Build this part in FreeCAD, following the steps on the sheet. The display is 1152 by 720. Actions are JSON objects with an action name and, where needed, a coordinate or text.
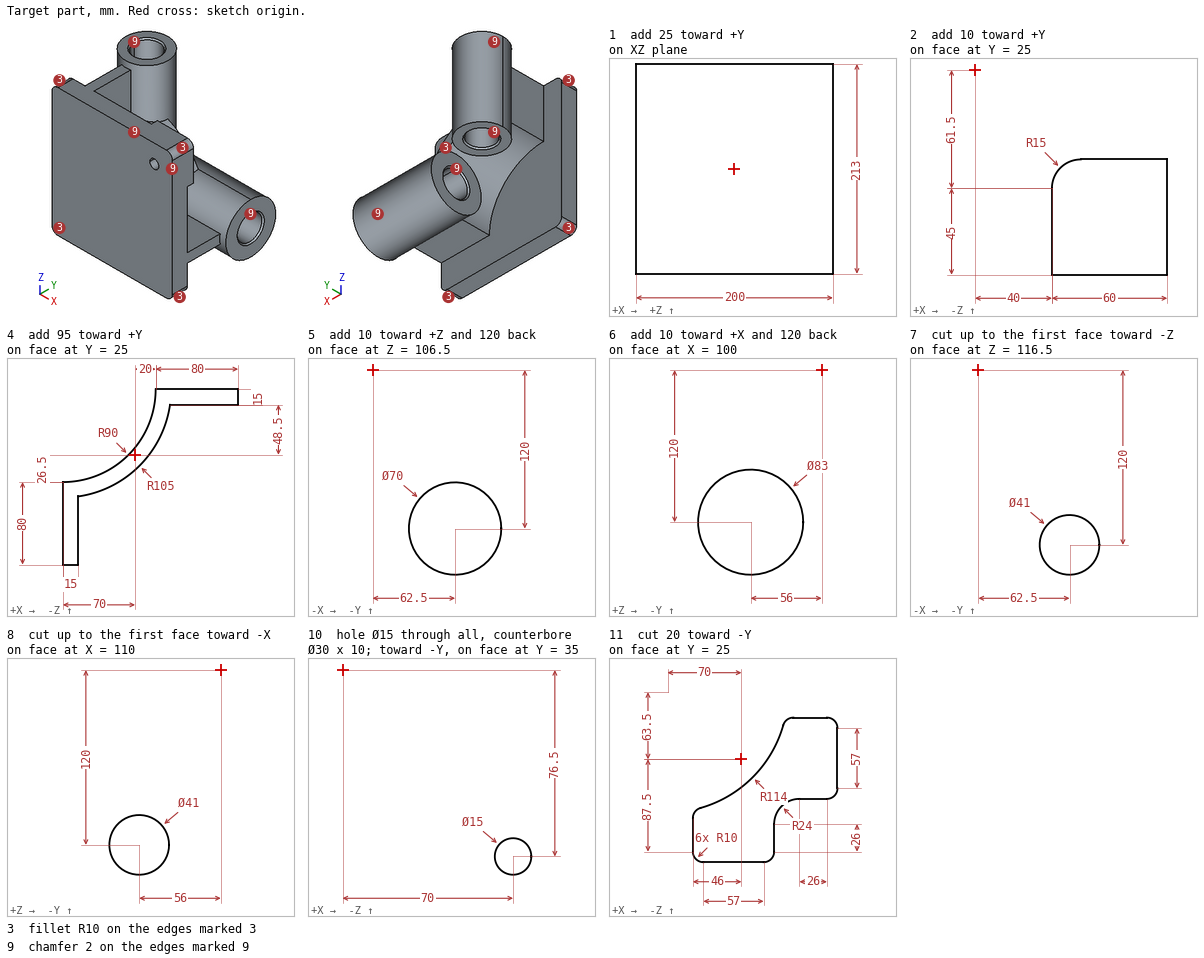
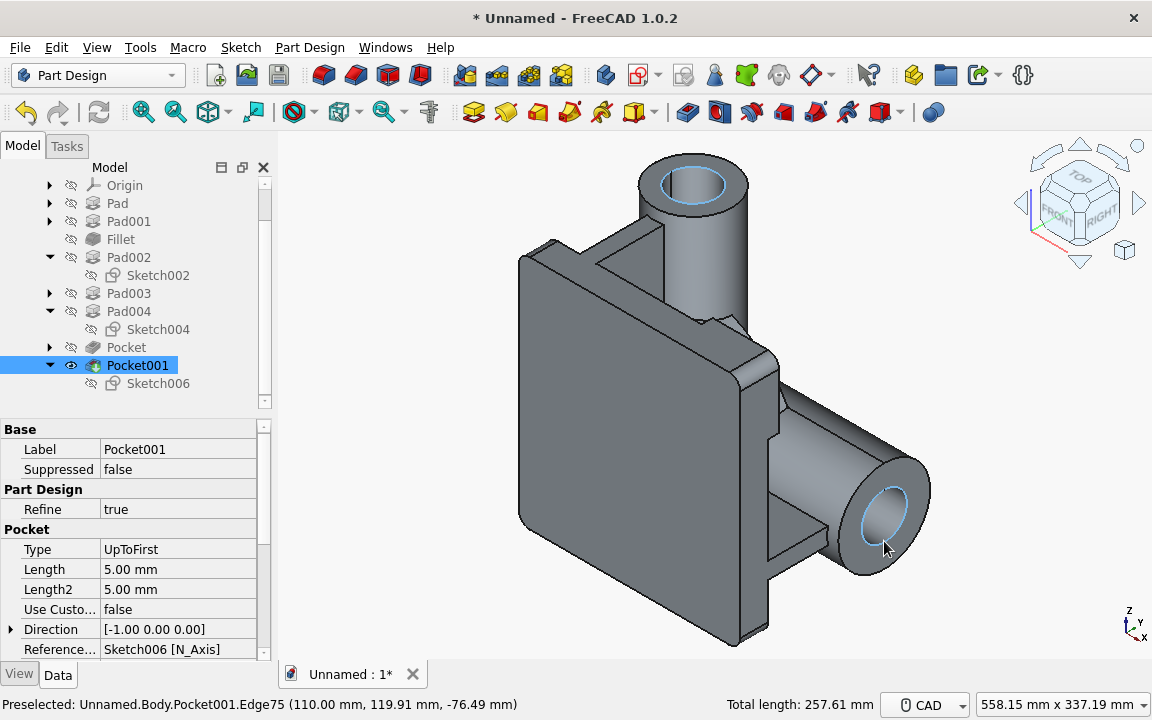
{"action": "key", "text": "2"}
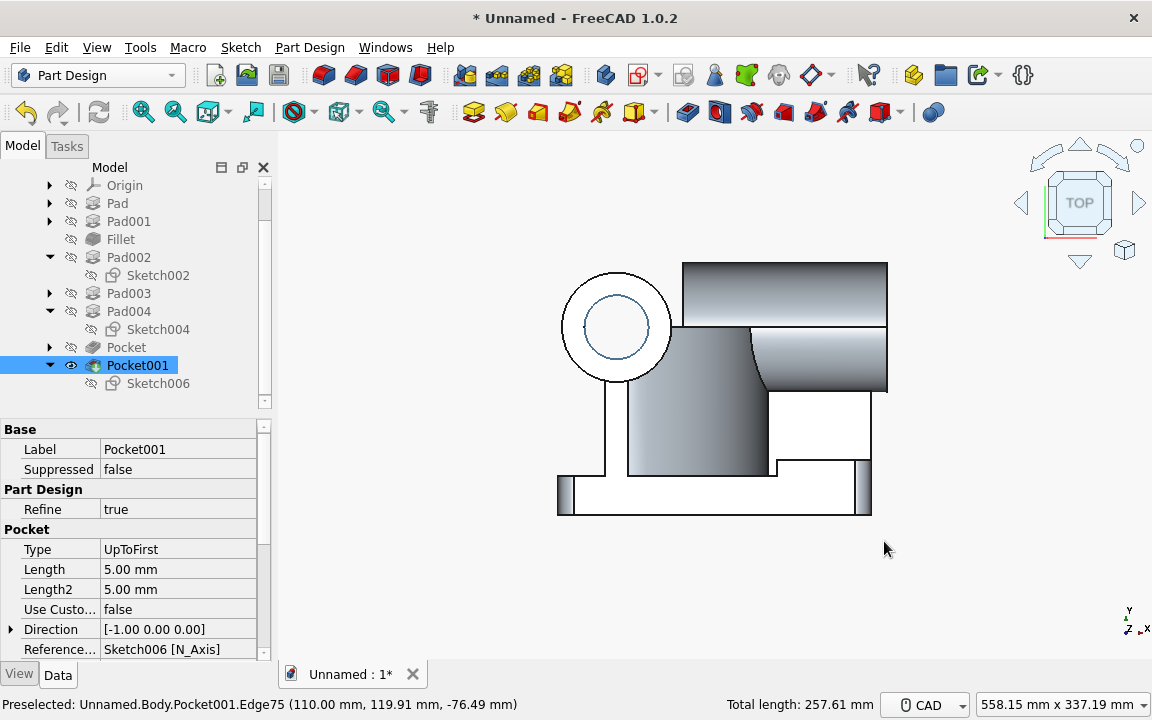
{"action": "key", "text": "0"}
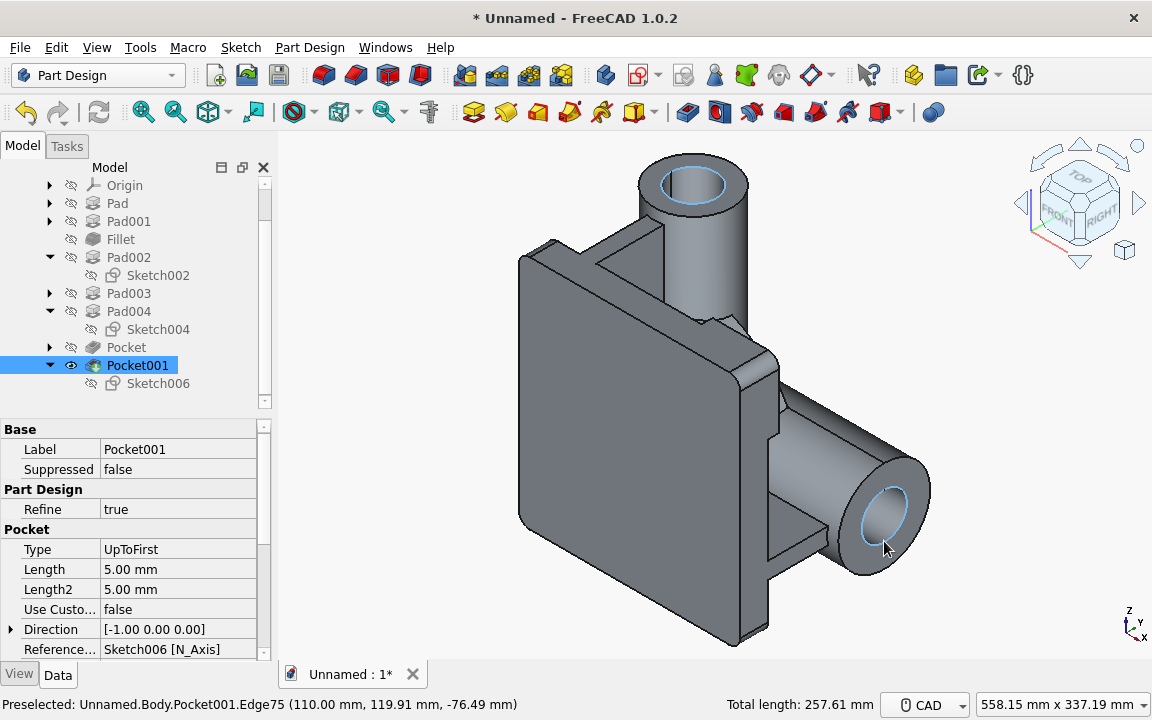
{"action": "key", "text": "1"}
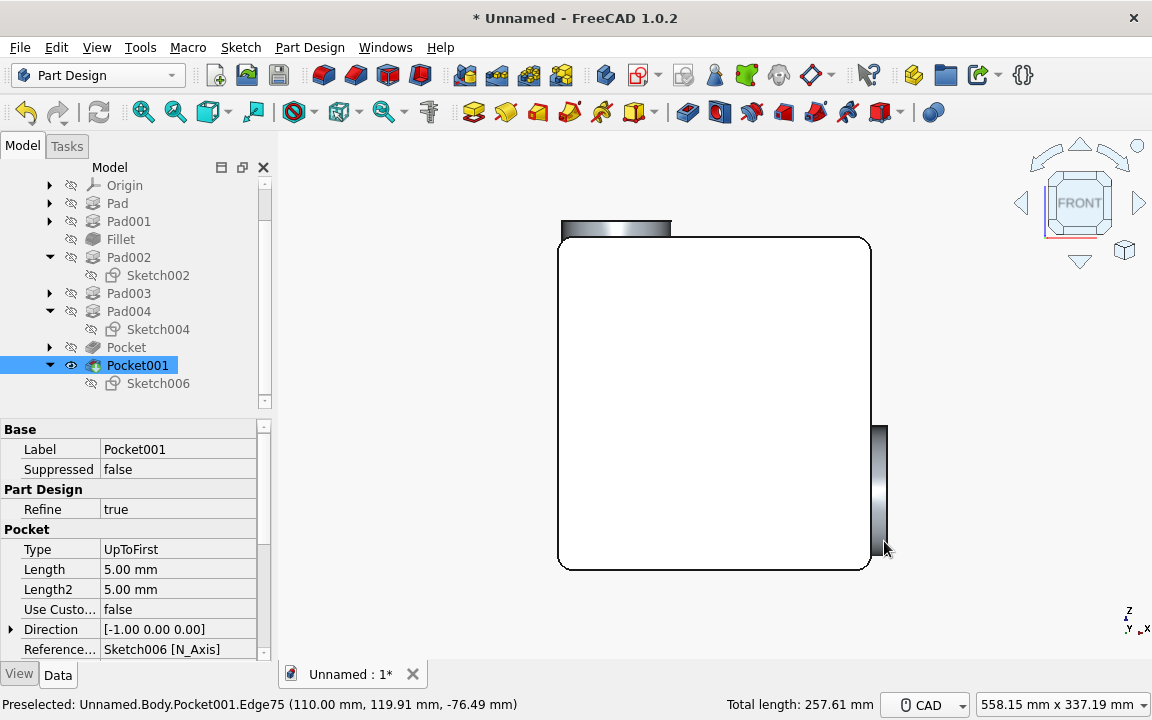
{"action": "key", "text": "3"}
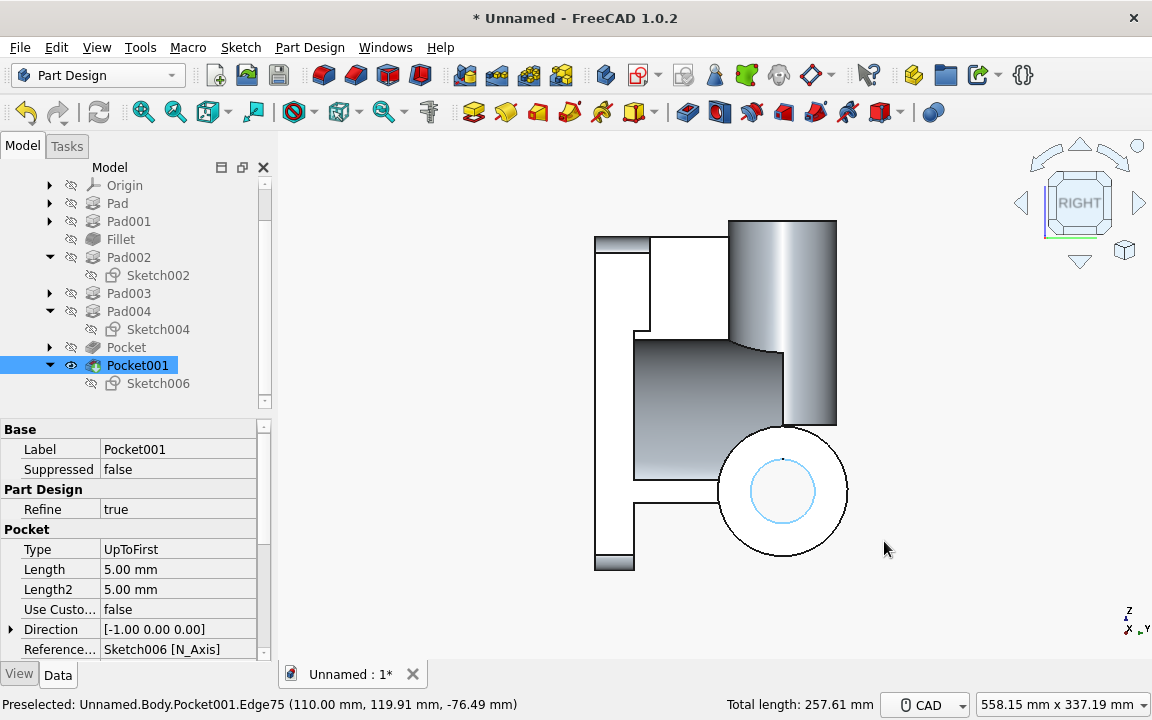
{"action": "key", "text": "5"}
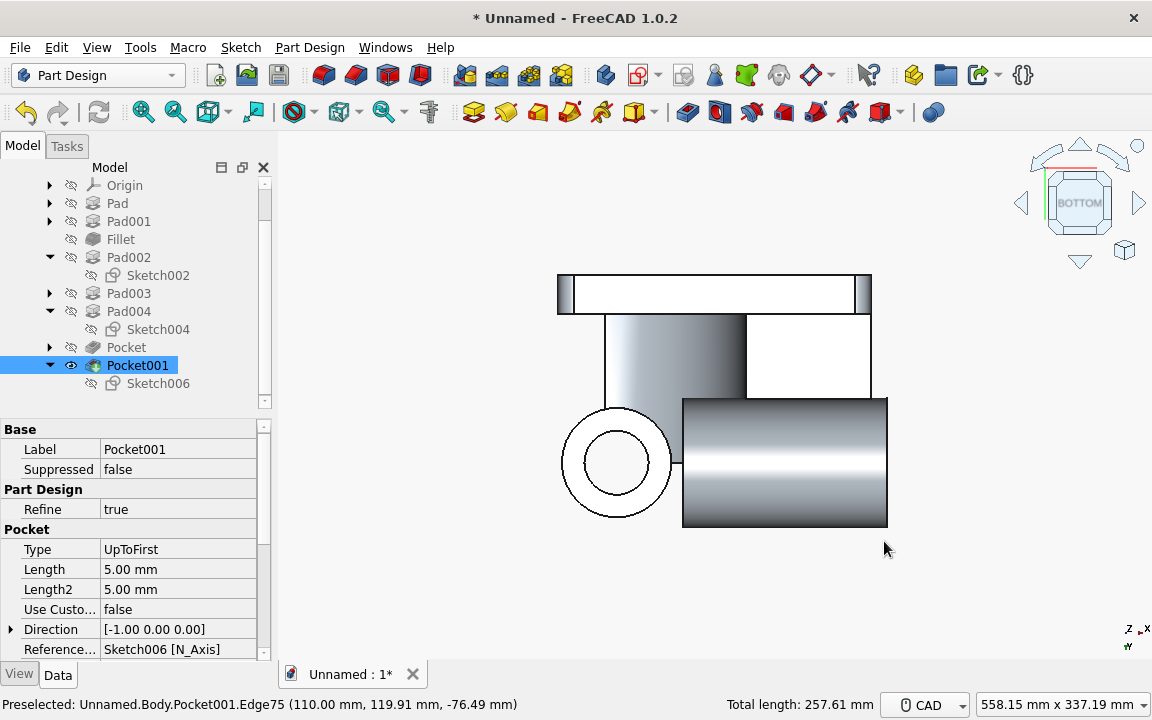
{"action": "left_click", "coordinate": [643, 443], "text": "ctrl"}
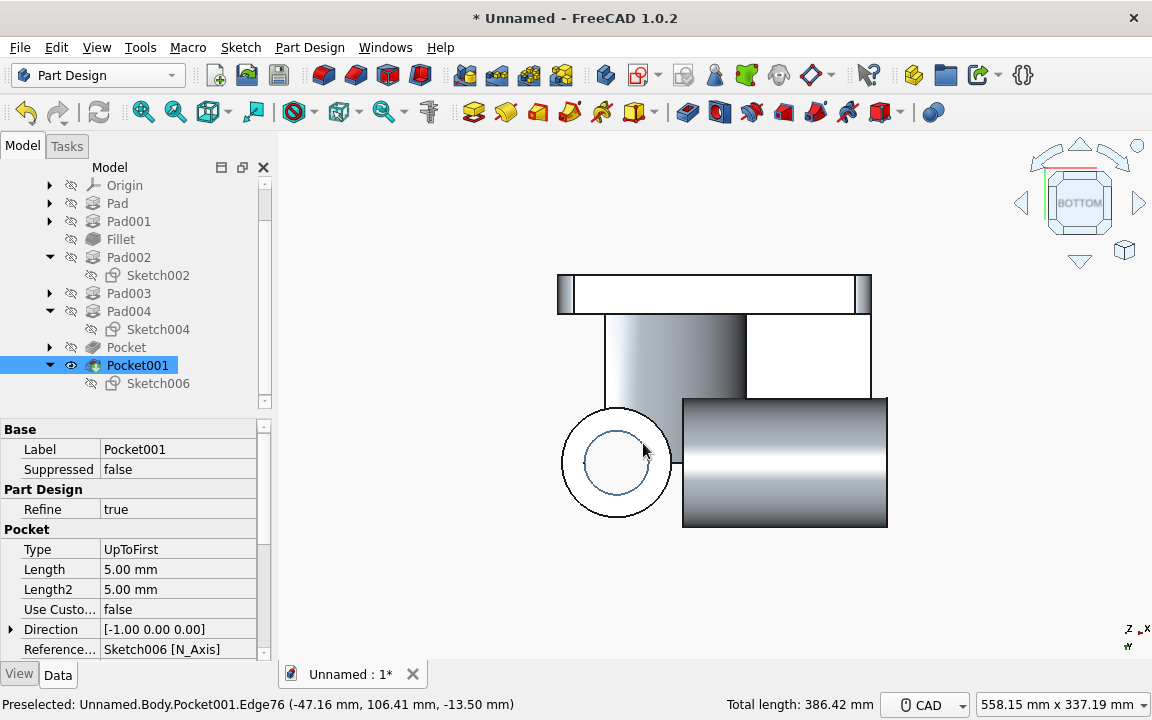
{"action": "key", "text": "4"}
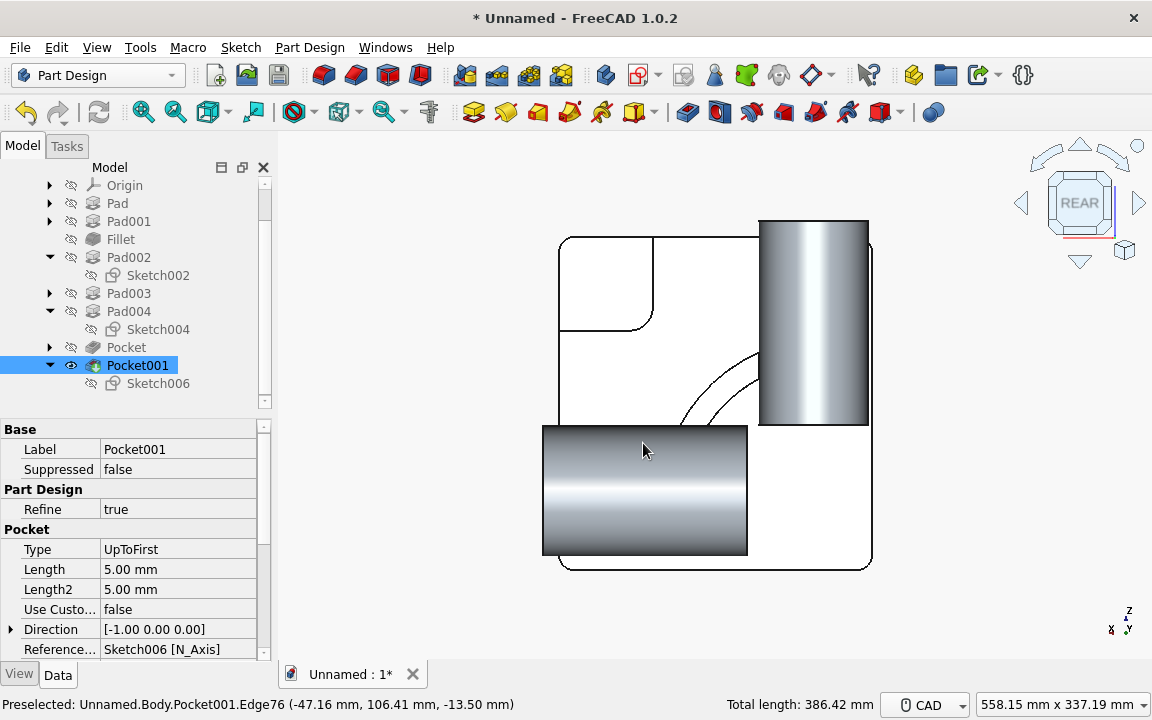
{"action": "key", "text": "6"}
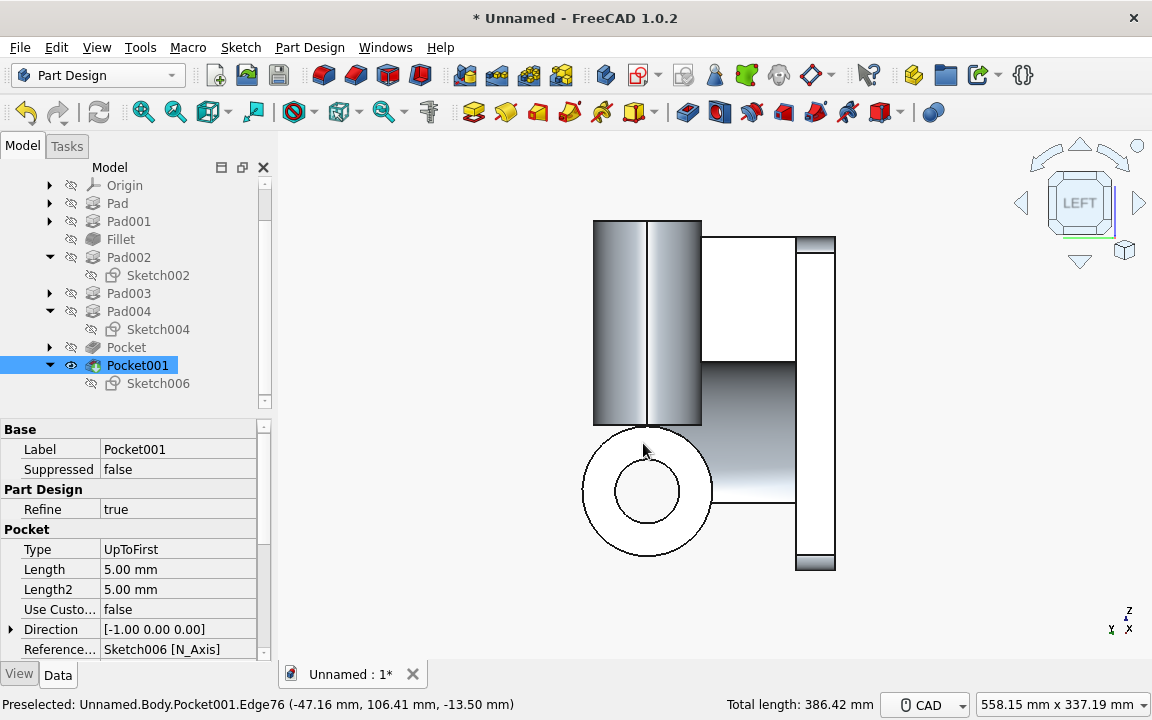
{"action": "left_click", "coordinate": [647, 522], "text": "ctrl"}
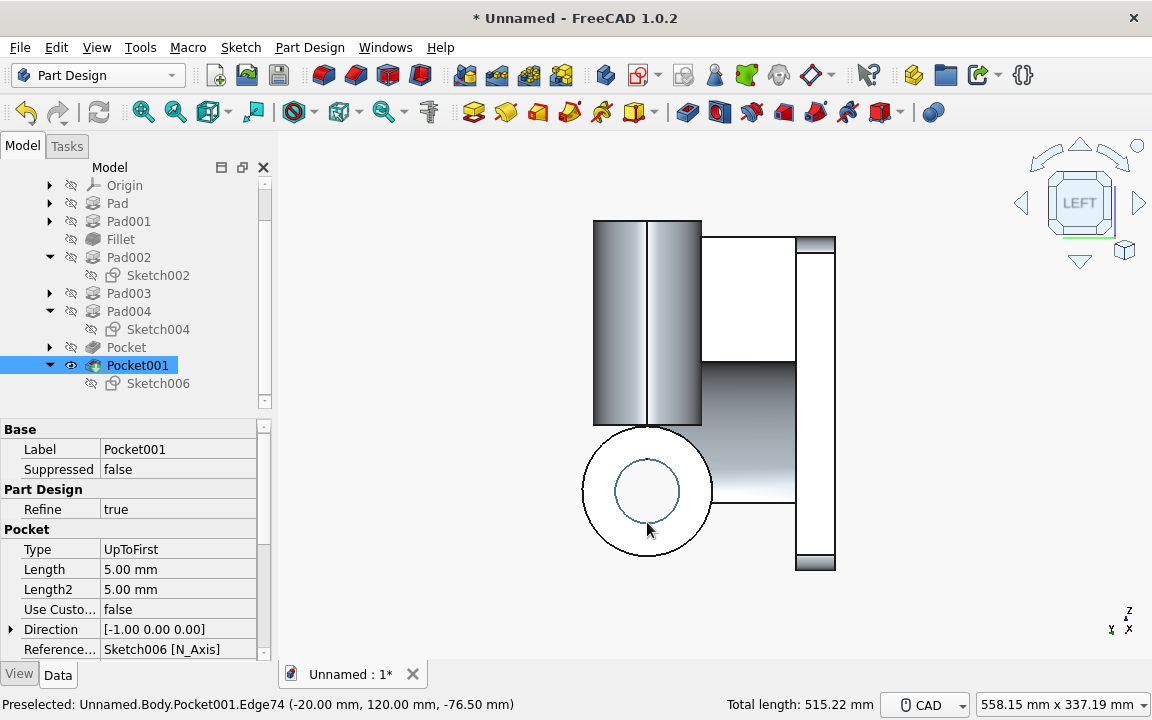
{"action": "left_click", "coordinate": [356, 76]}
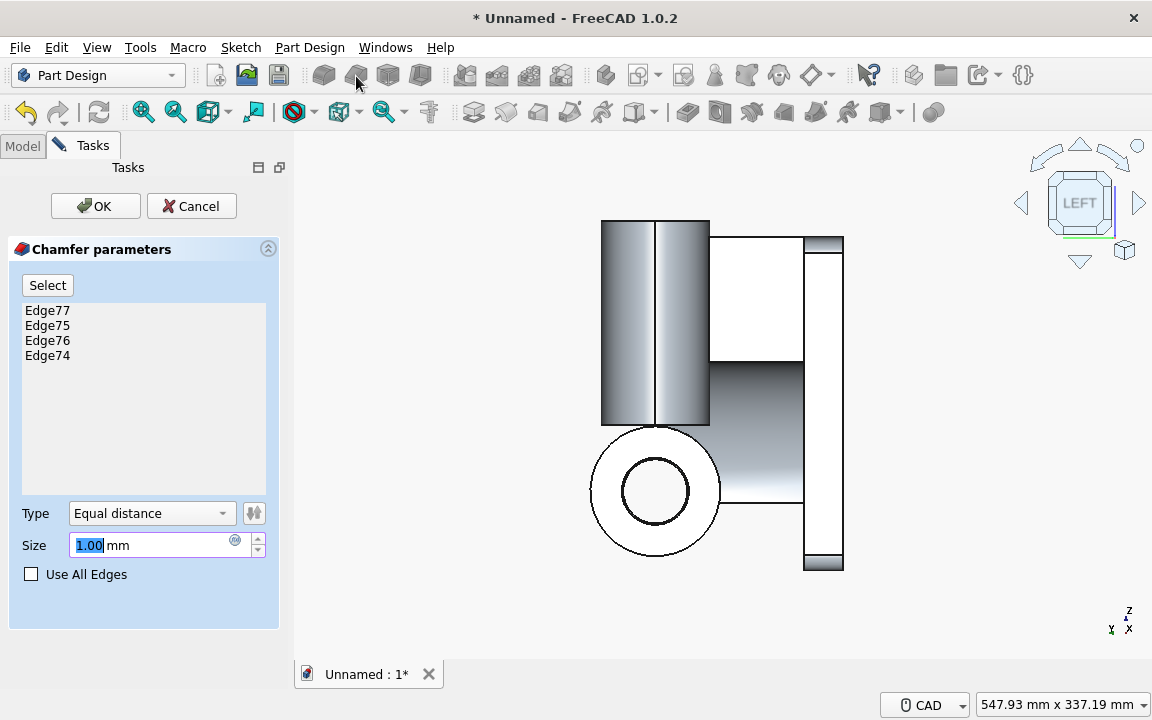
{"action": "type", "text": "2"}
{"action": "key", "text": "Tab"}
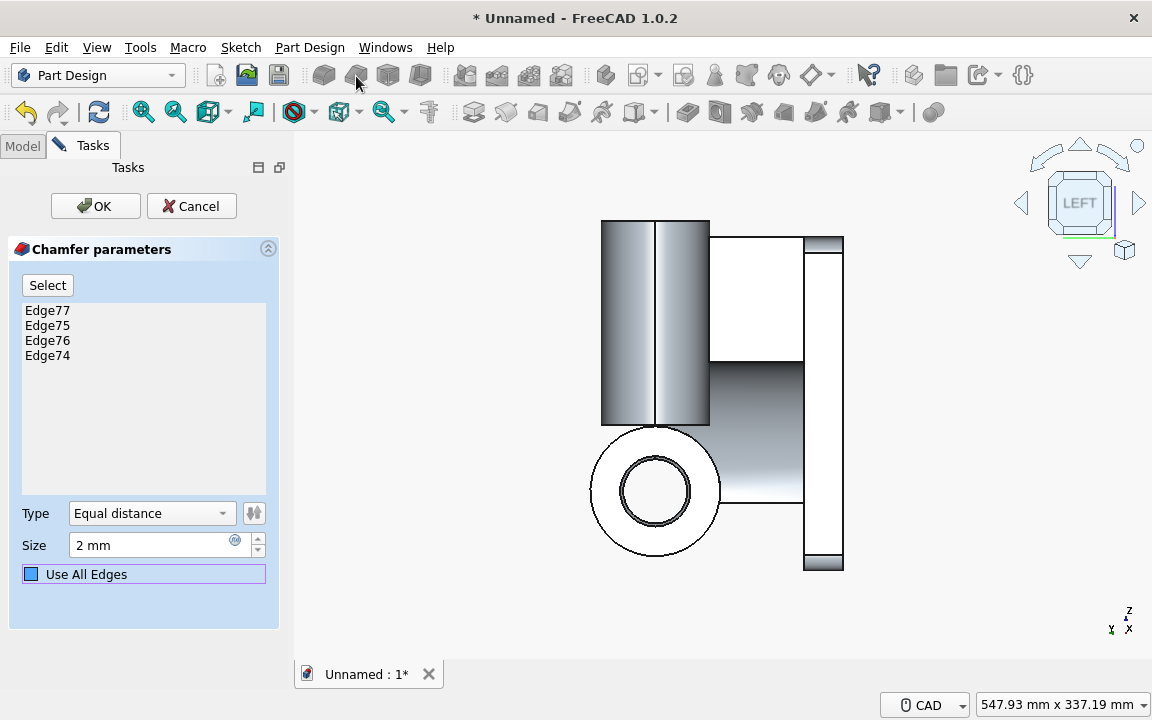
{"action": "left_click", "coordinate": [96, 206]}